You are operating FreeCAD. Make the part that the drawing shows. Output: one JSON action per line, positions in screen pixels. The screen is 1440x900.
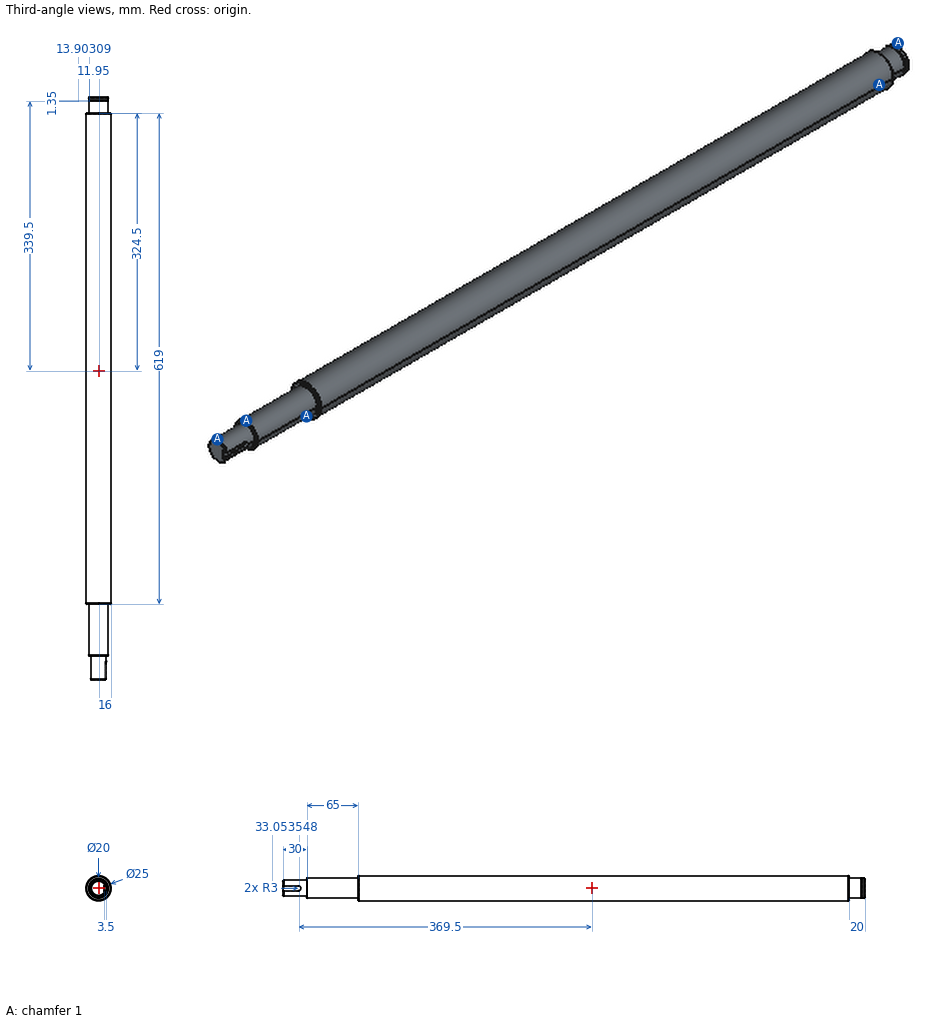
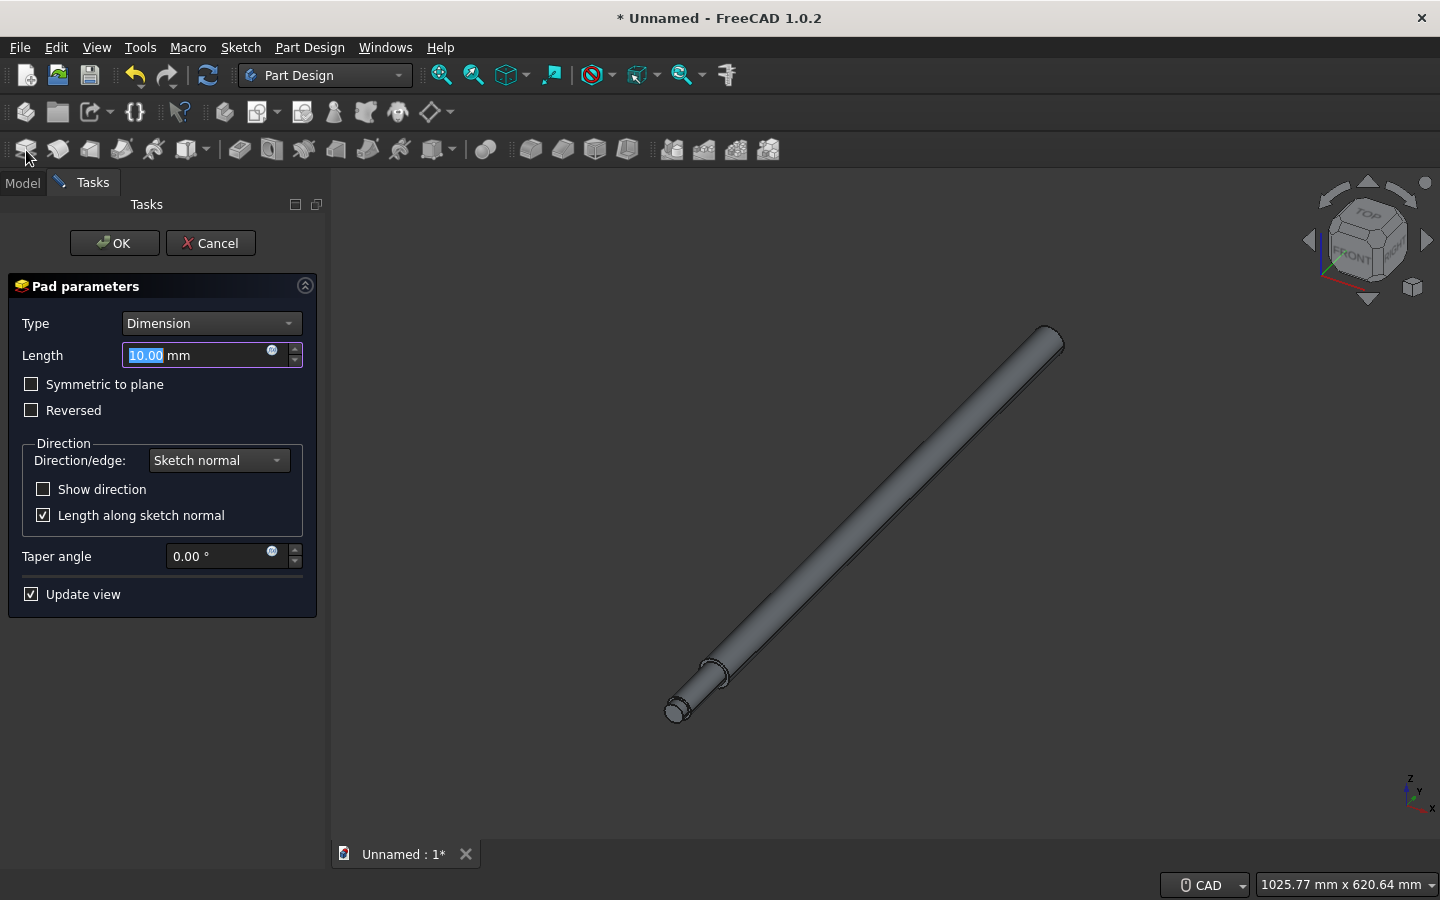
{"action": "type", "text": "30"}
{"action": "key", "text": "Tab"}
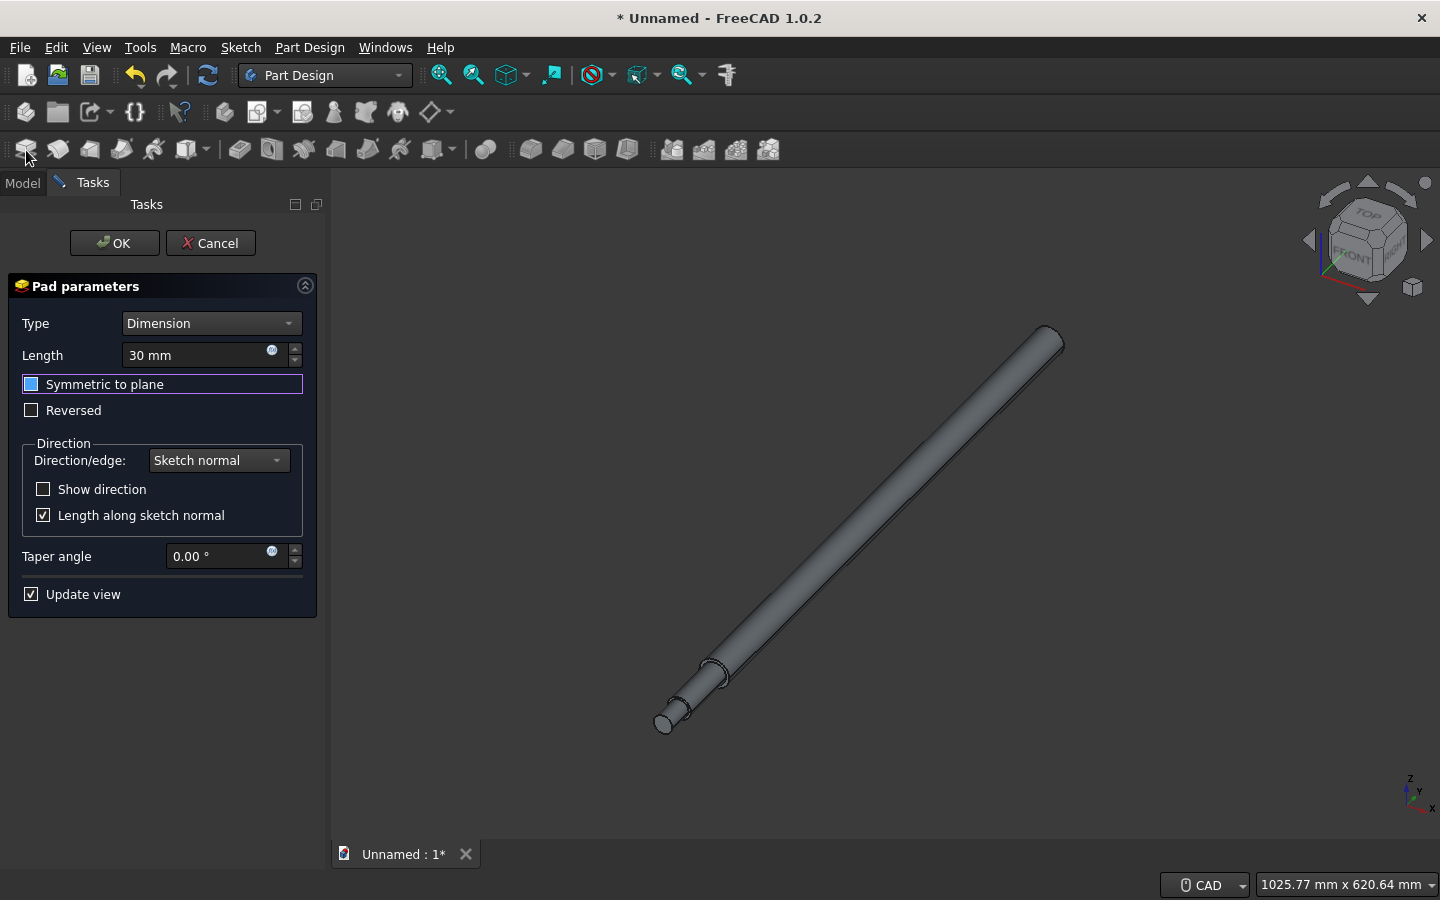
{"action": "left_click", "coordinate": [115, 243]}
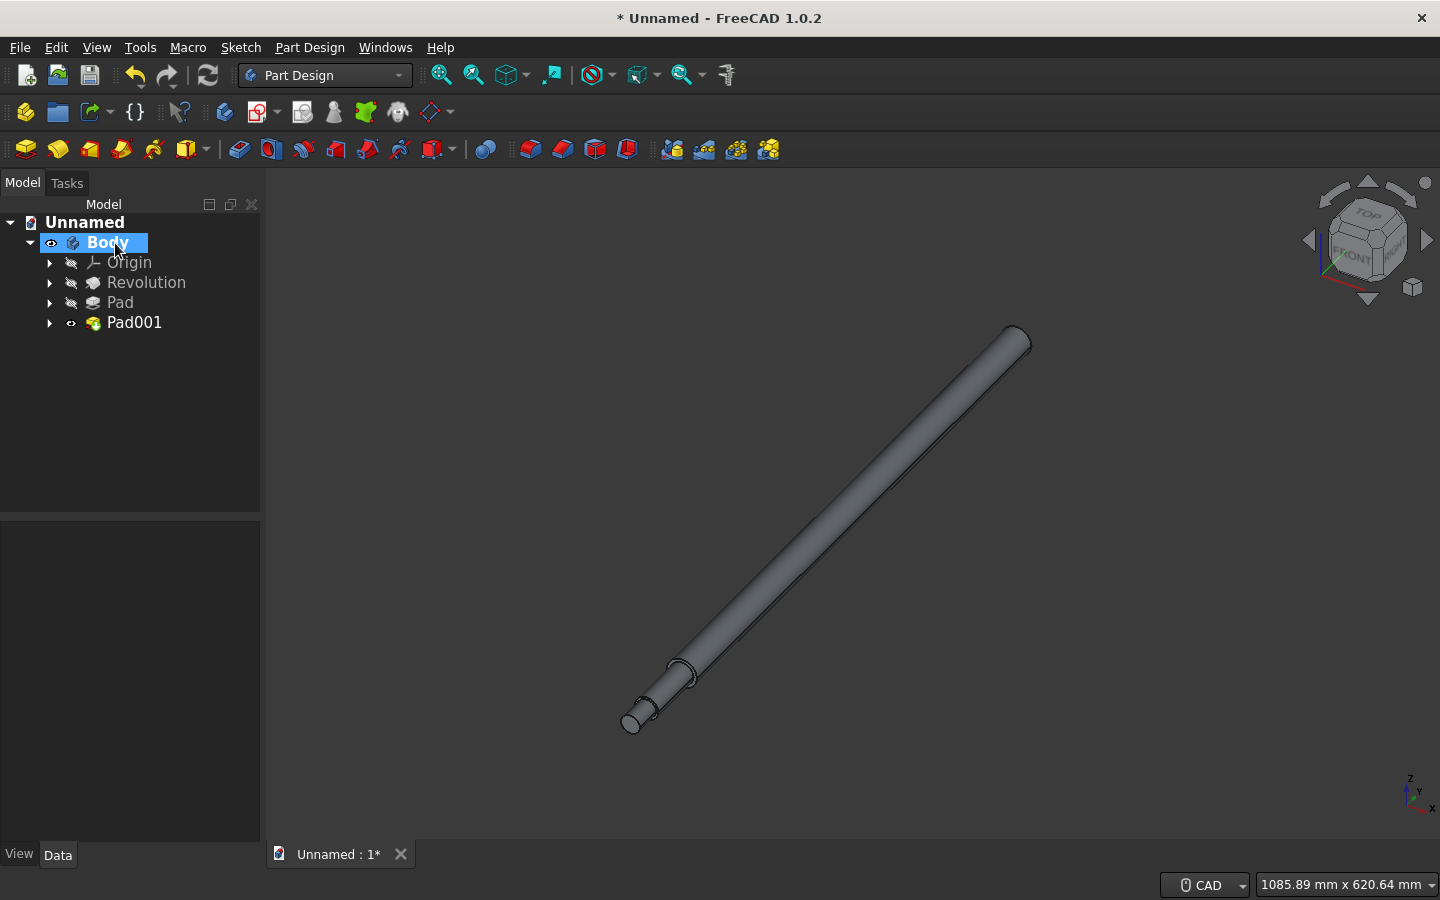
{"action": "left_click", "coordinate": [50, 263]}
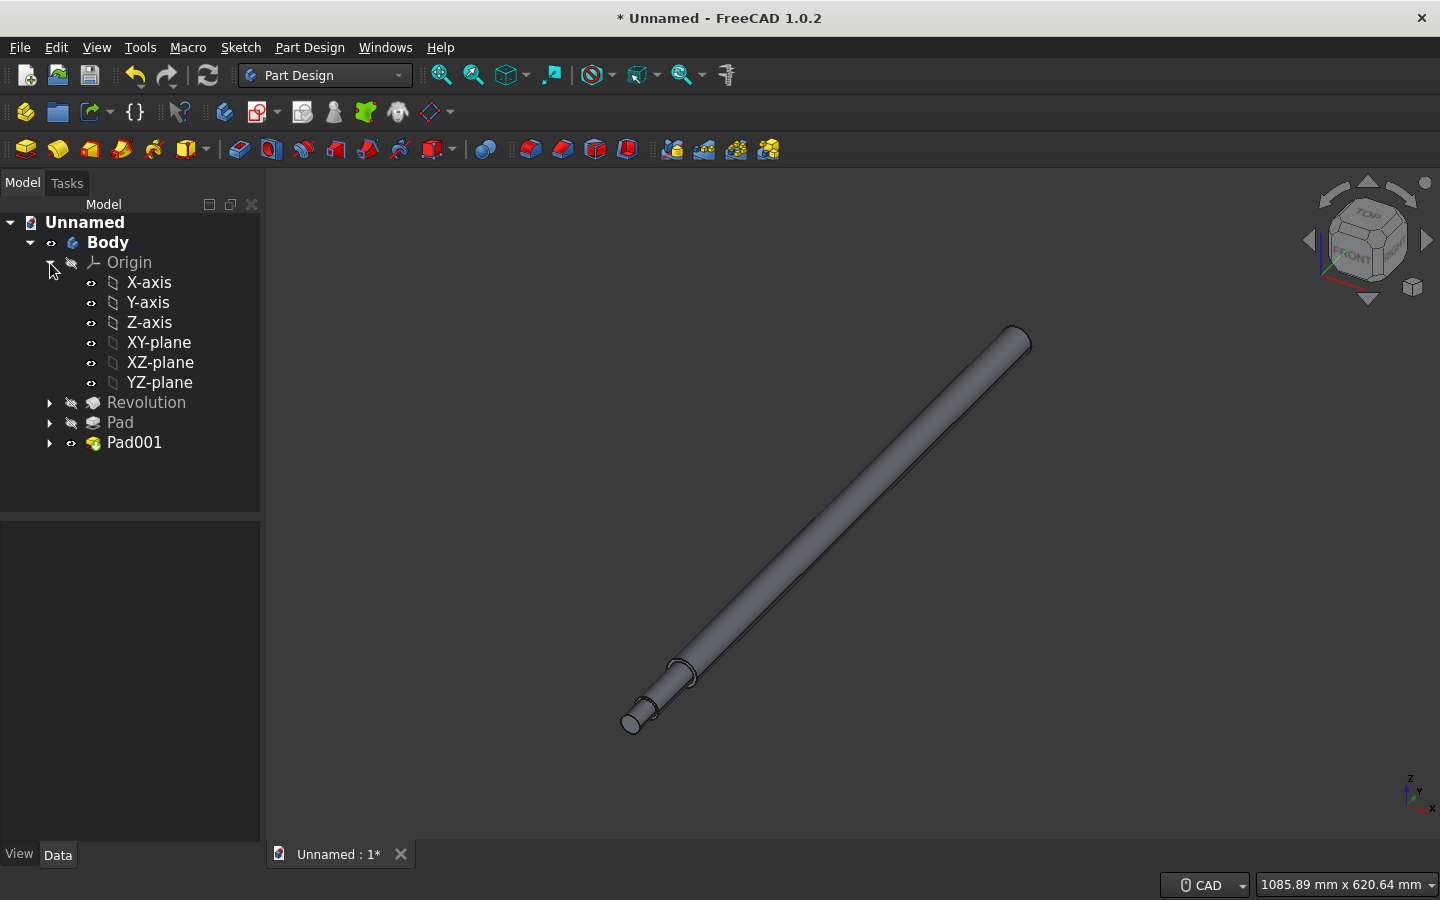
{"action": "left_click", "coordinate": [136, 363]}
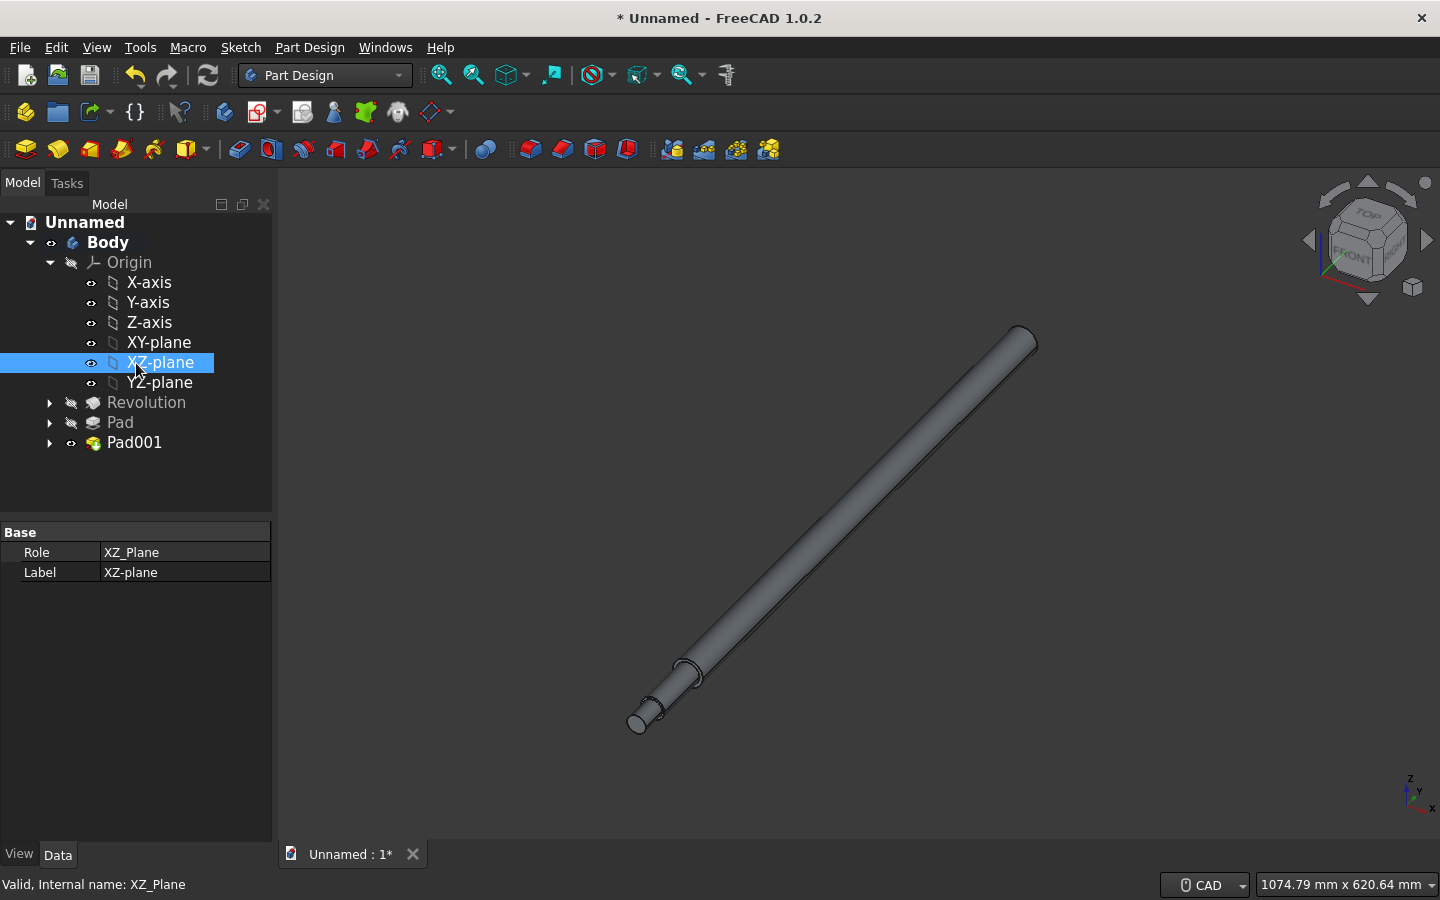
{"action": "left_click", "coordinate": [430, 112]}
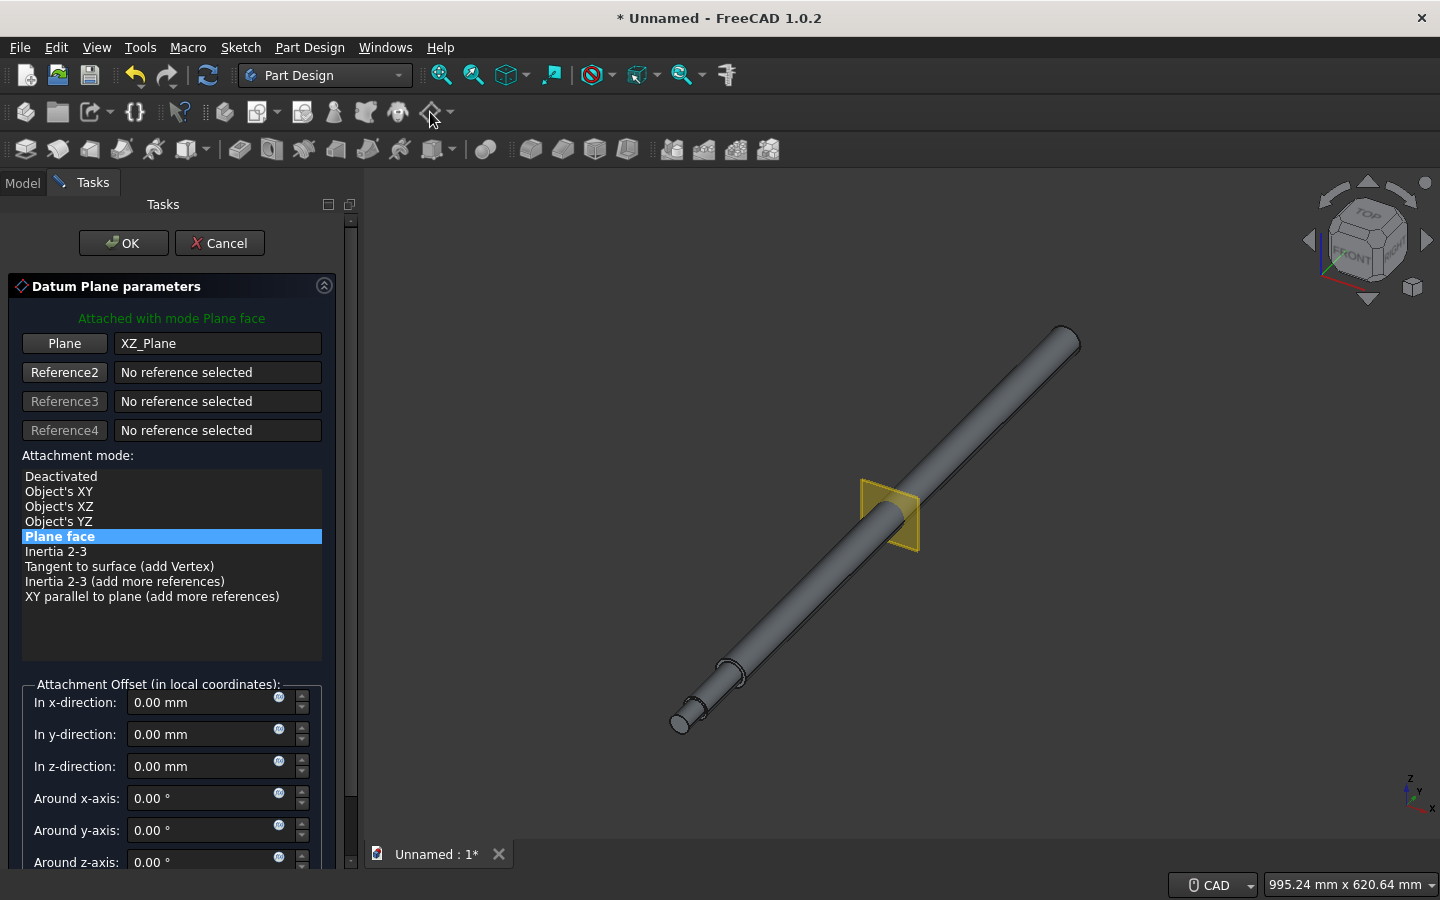
{"action": "triple_click", "coordinate": [210, 766]}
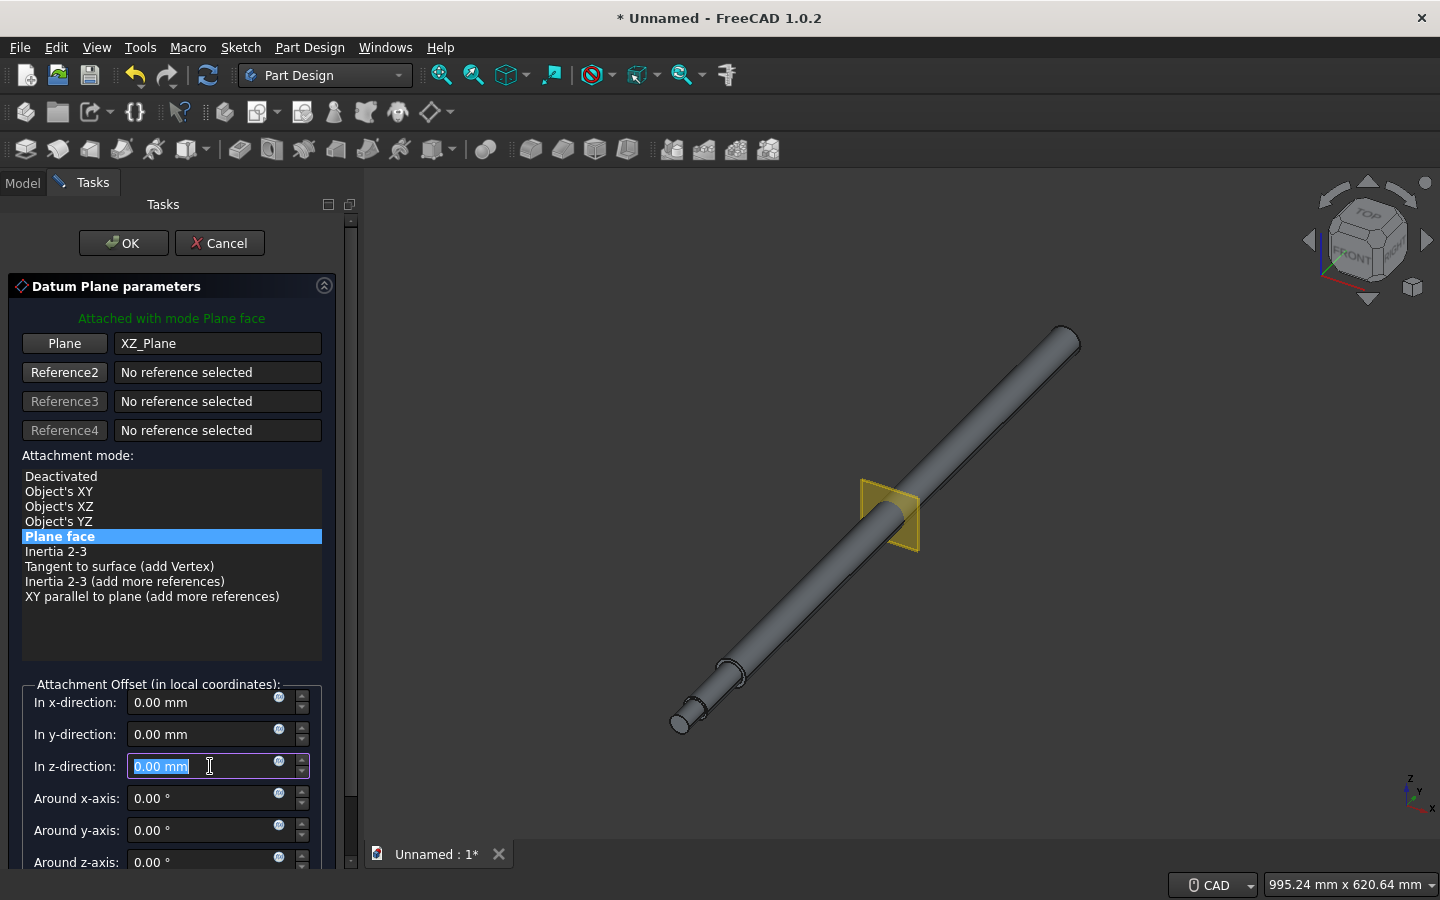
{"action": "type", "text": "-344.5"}
{"action": "key", "text": "Tab"}